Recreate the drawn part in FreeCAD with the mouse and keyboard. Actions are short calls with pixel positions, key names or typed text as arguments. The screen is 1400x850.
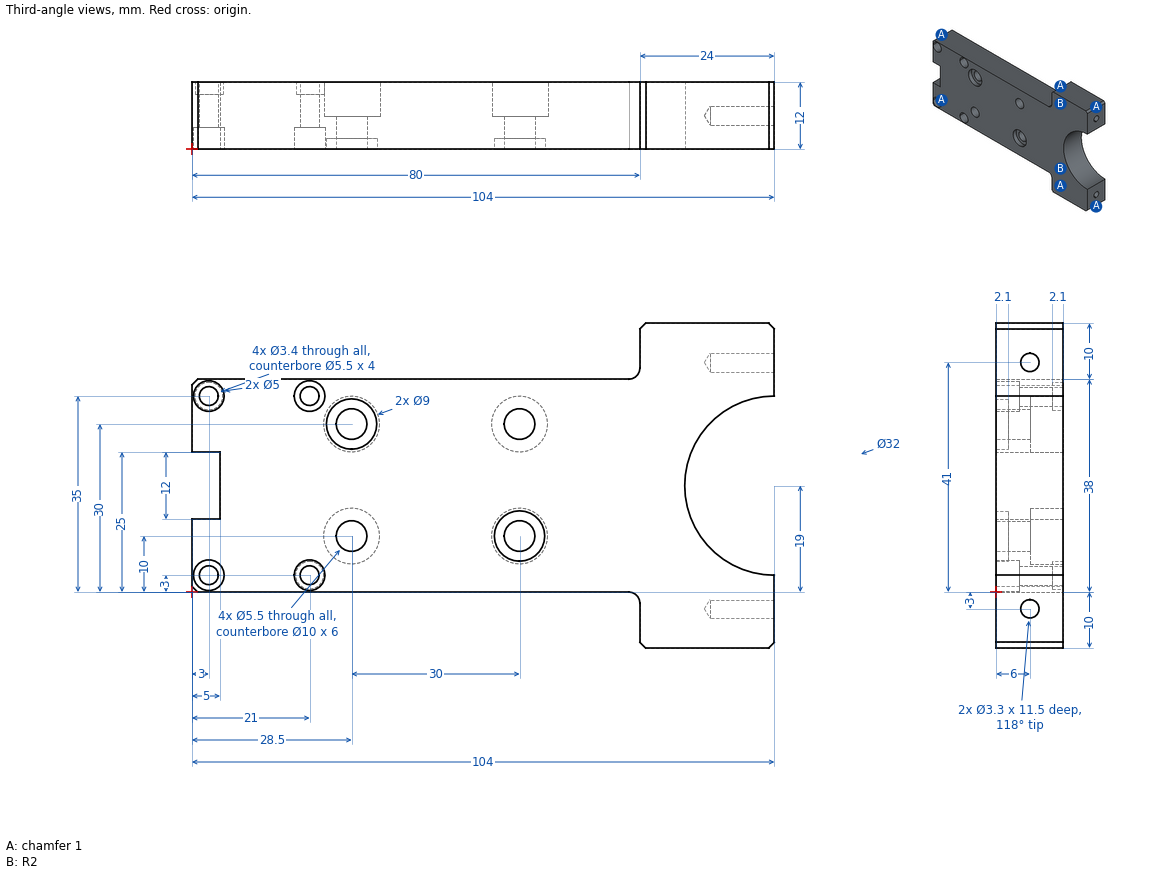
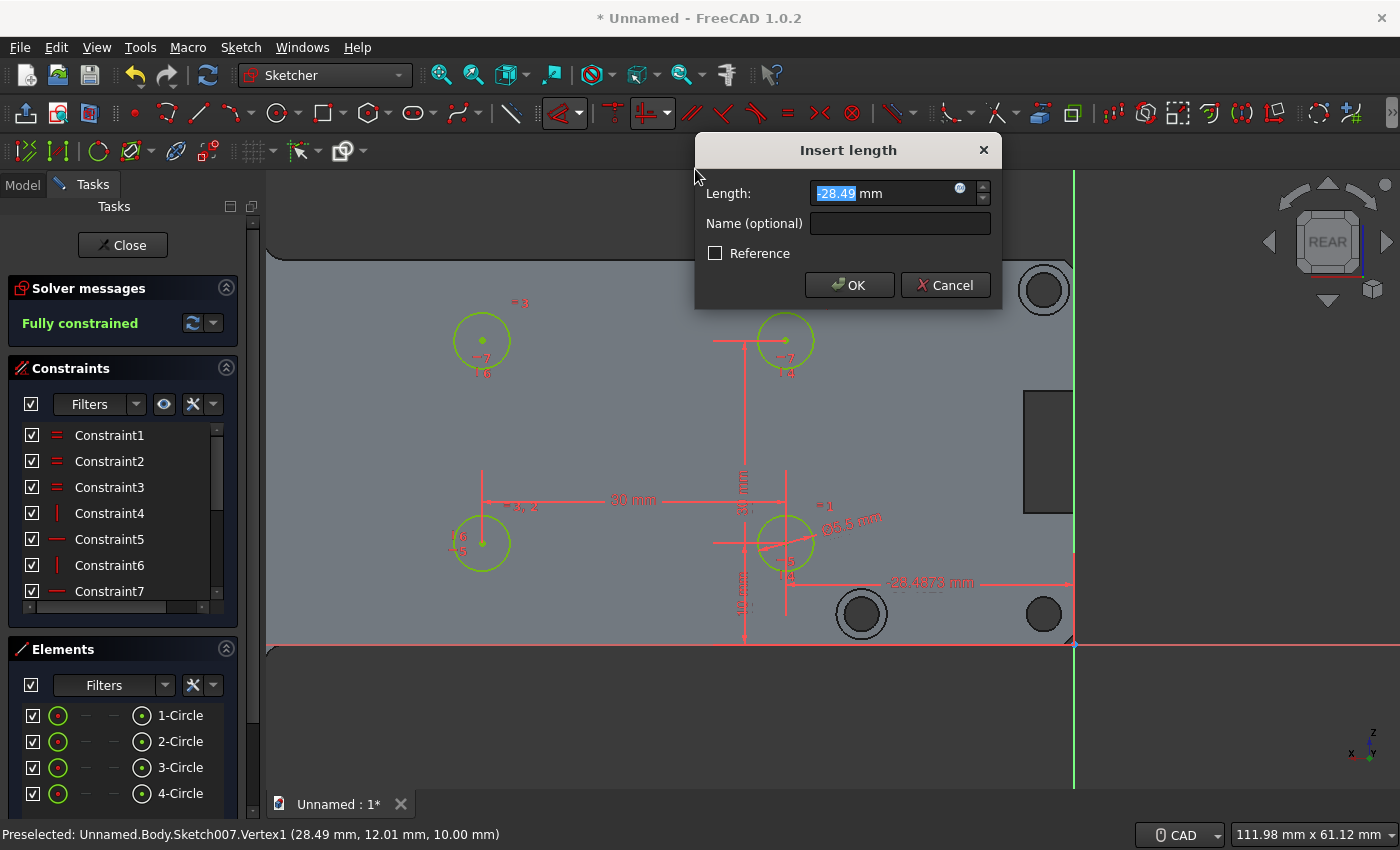
text(-28.5)
key(Return)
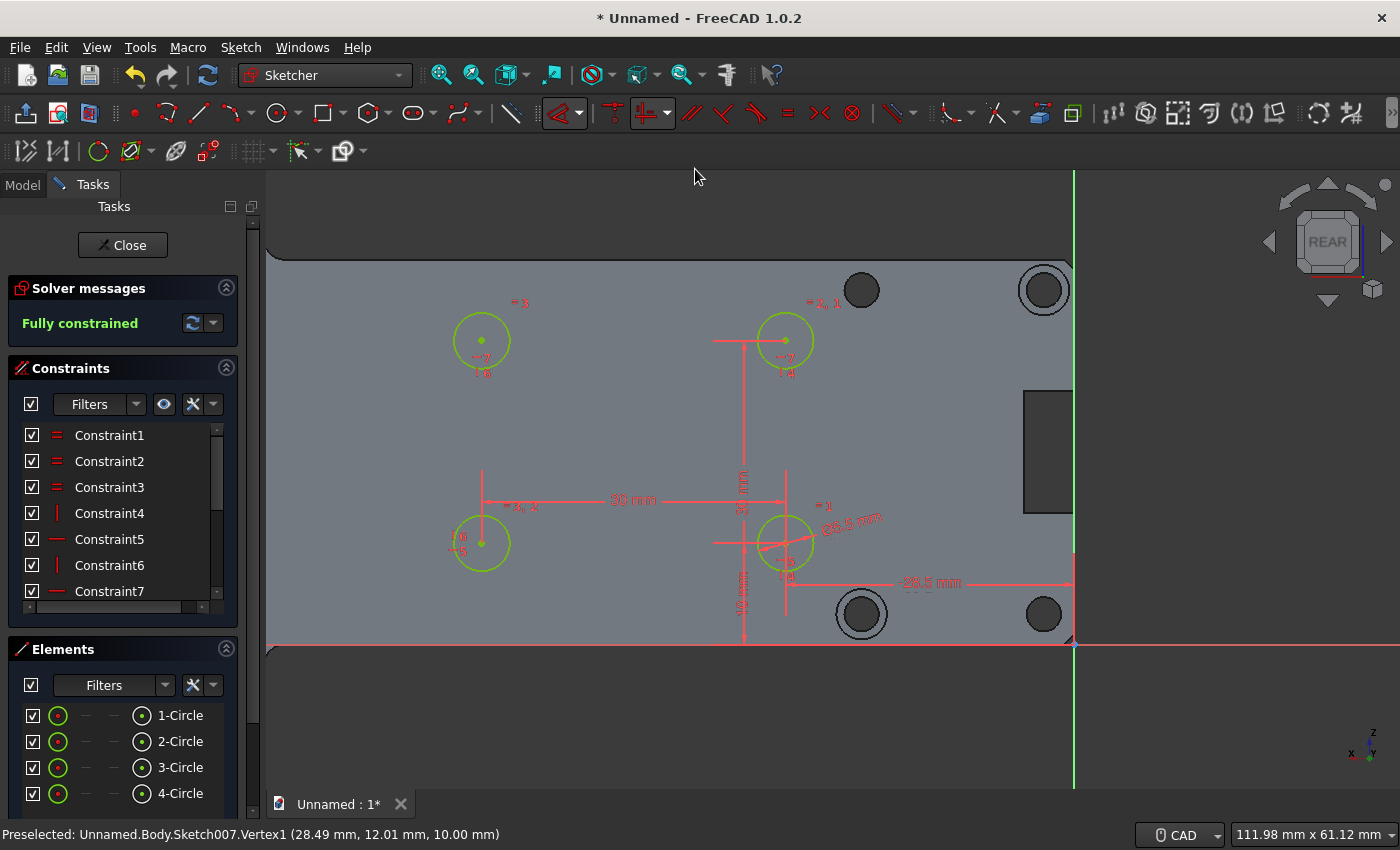
click(123, 245)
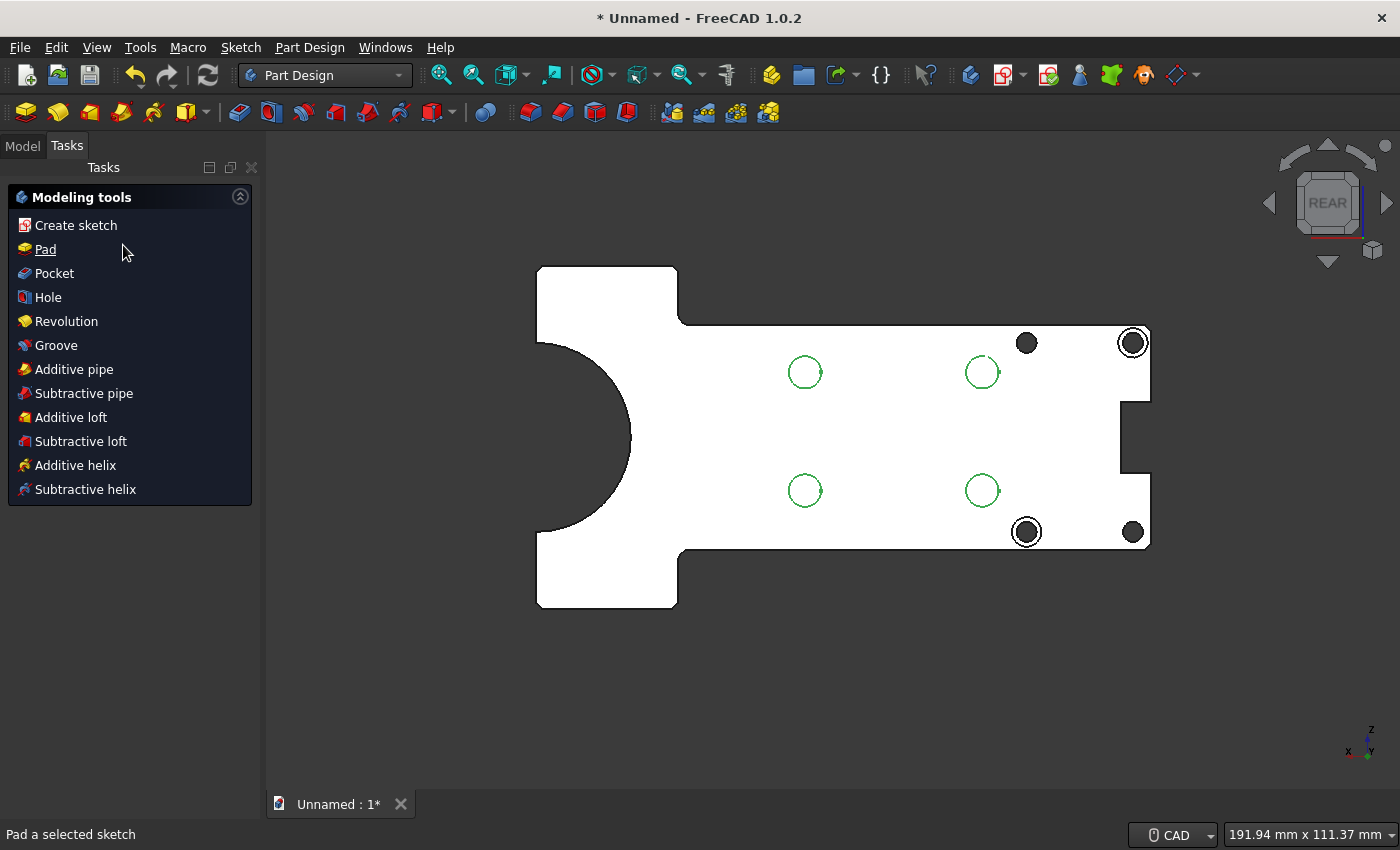
click(272, 112)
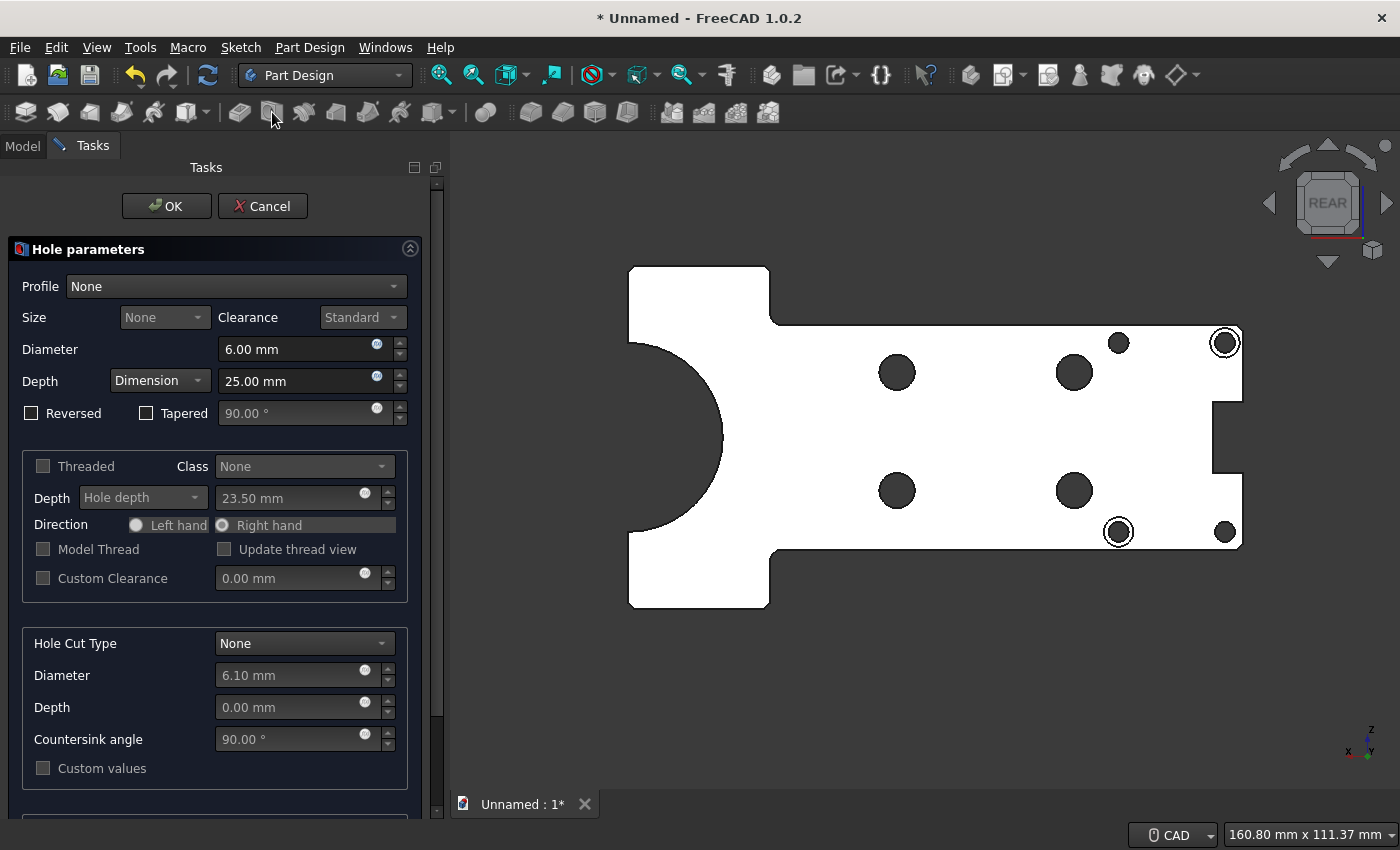
triple_click(305, 349)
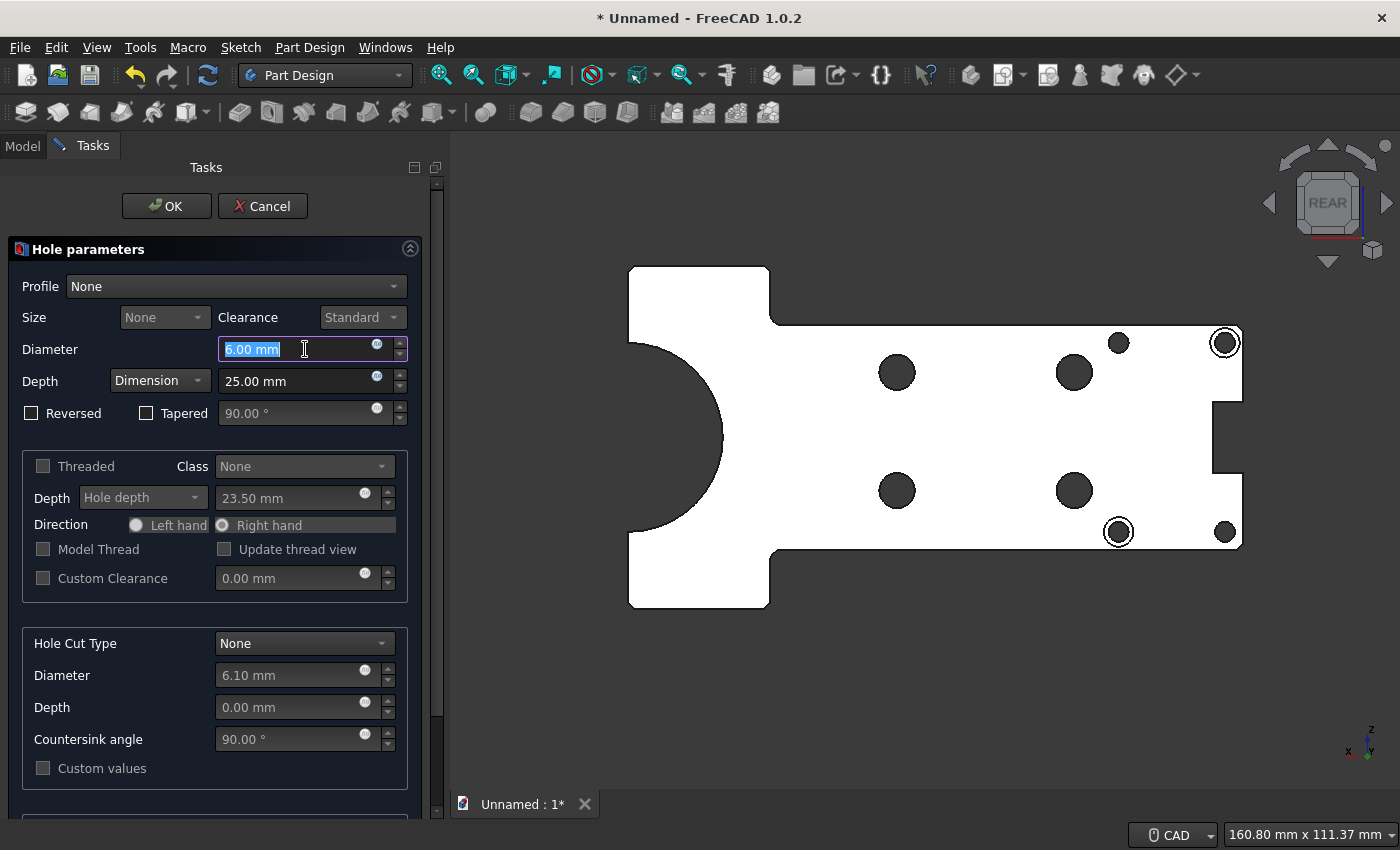
text(5.5)
key(Tab)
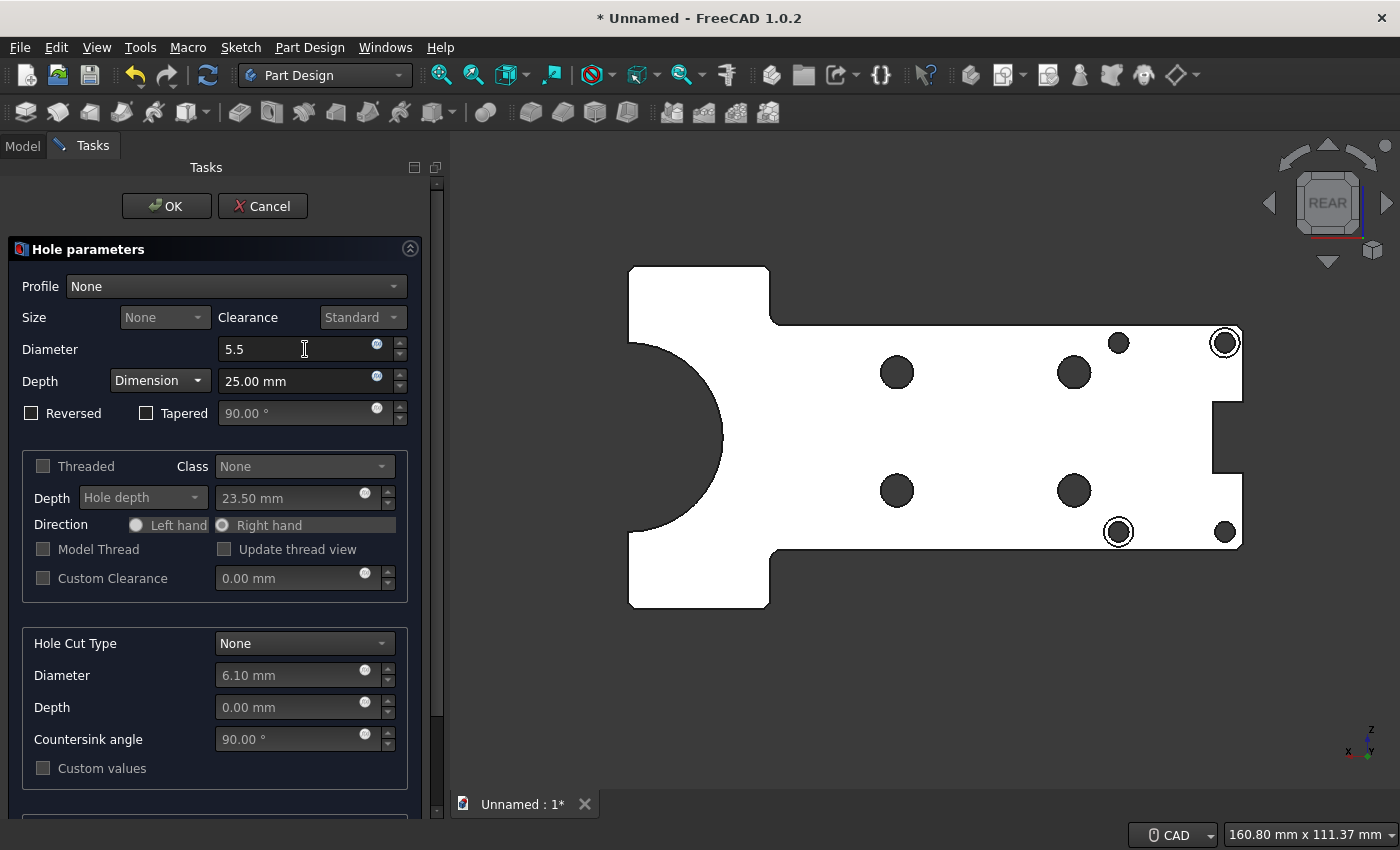
click(161, 380)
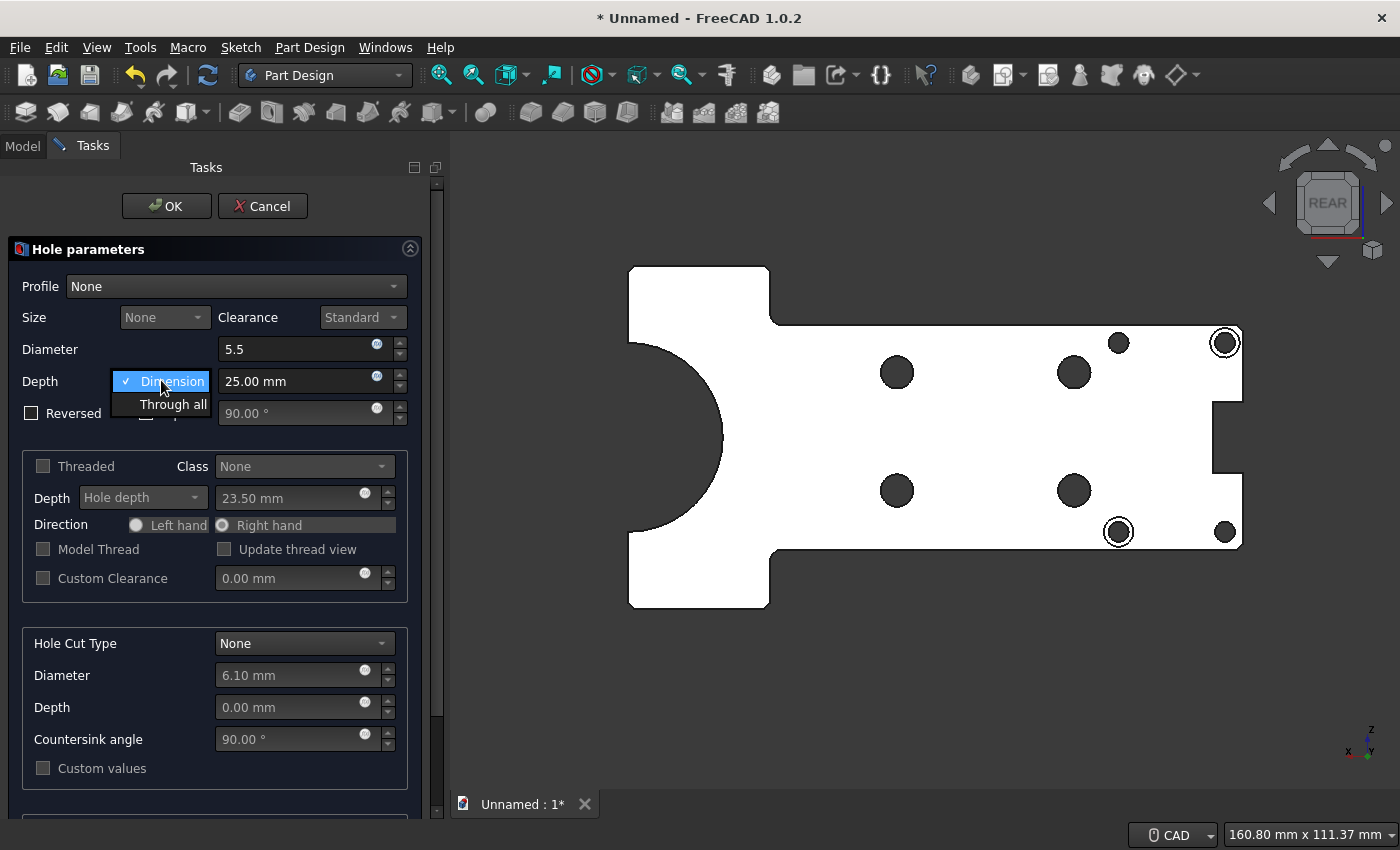
click(160, 404)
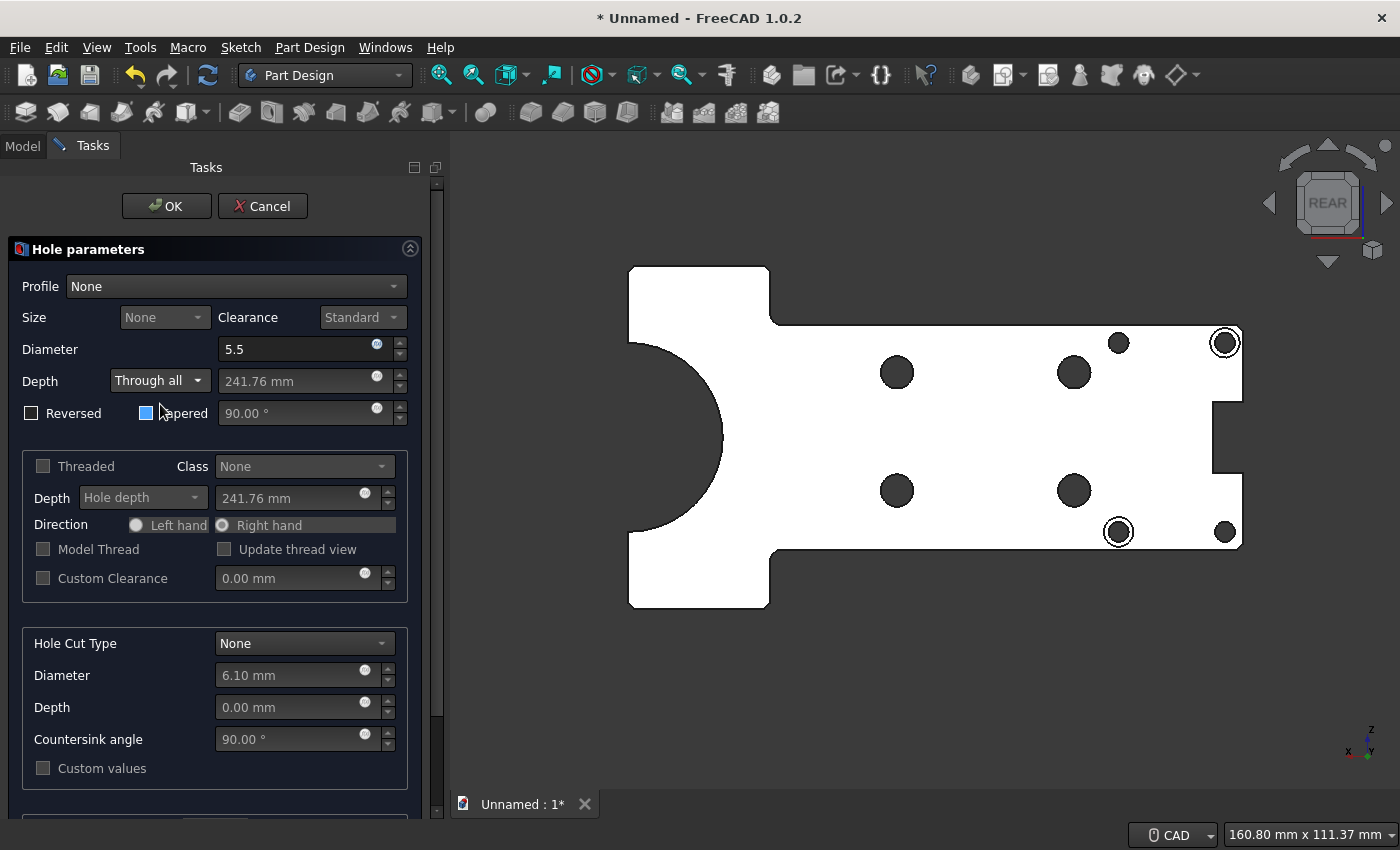
click(306, 644)